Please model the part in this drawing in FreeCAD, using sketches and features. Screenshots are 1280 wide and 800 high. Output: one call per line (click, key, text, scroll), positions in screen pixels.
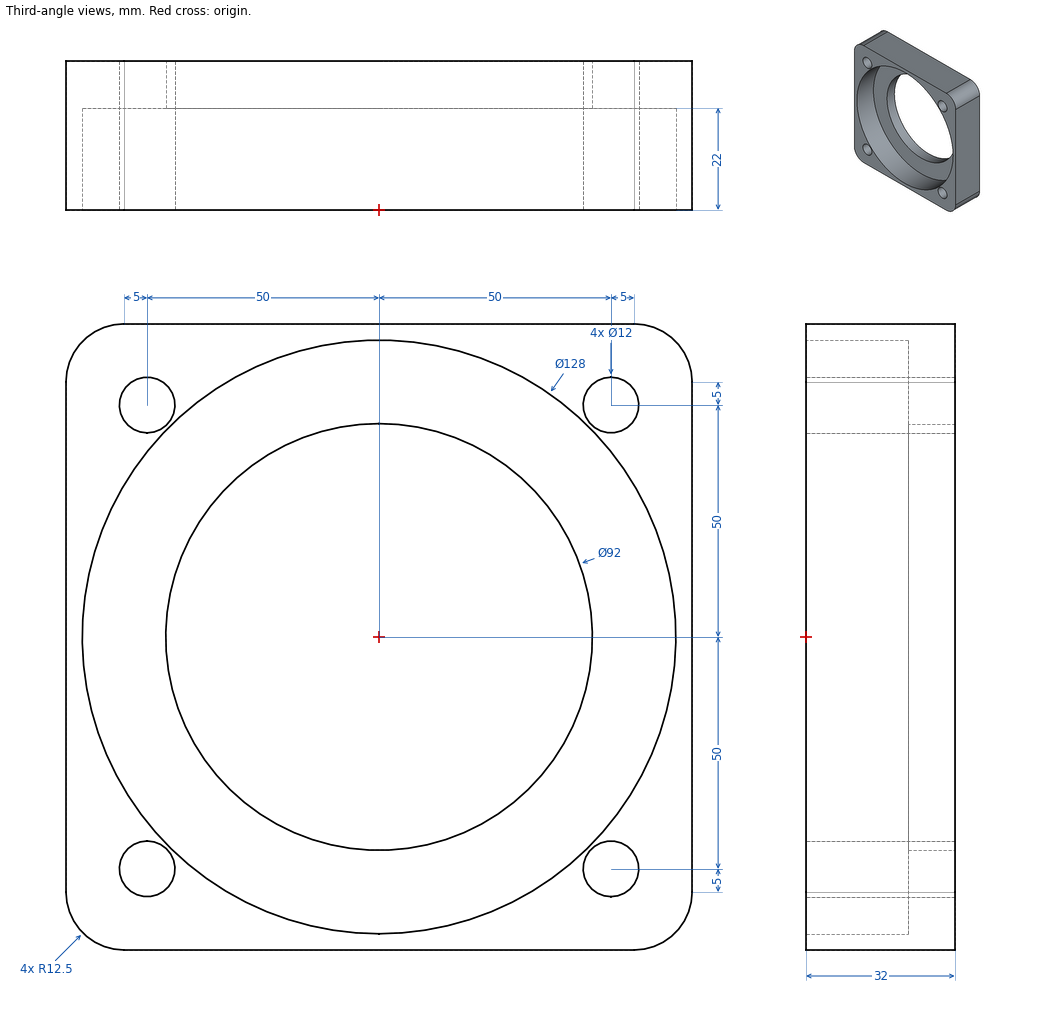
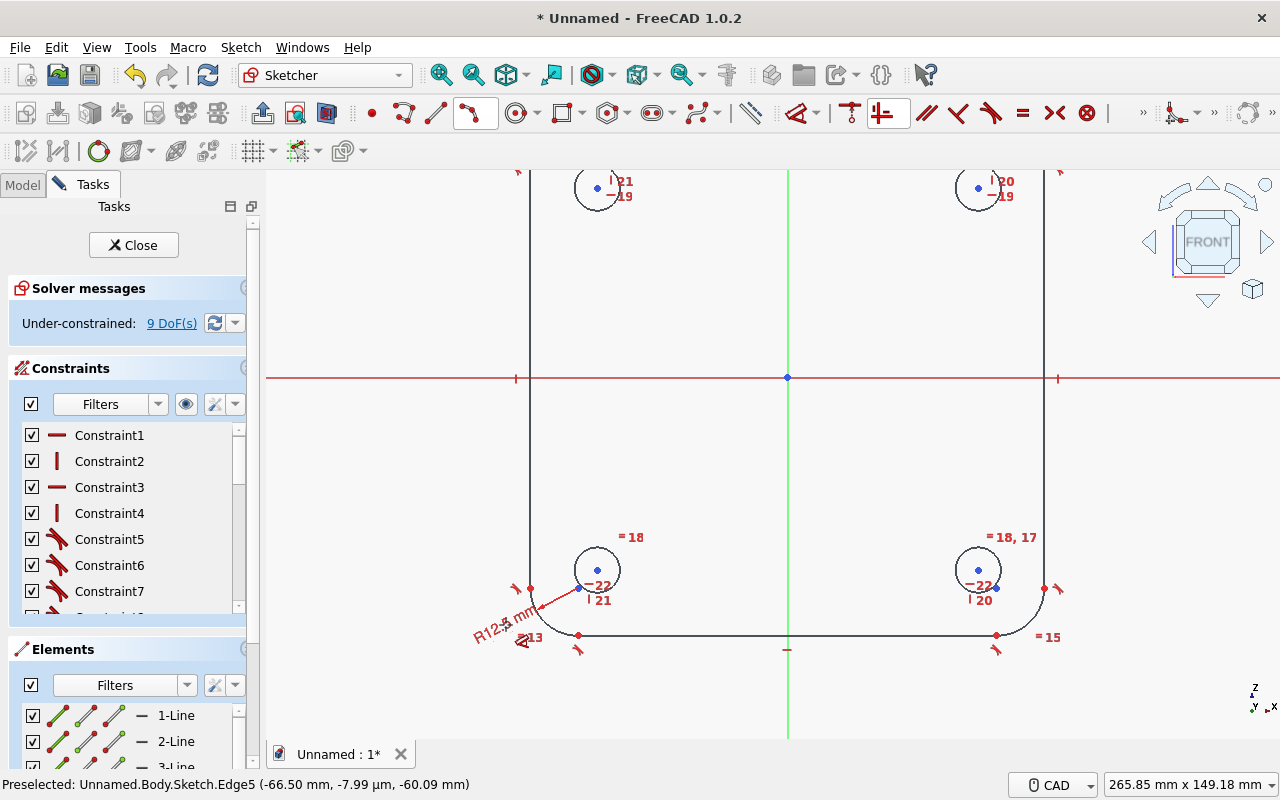
click(962, 204)
click(939, 226)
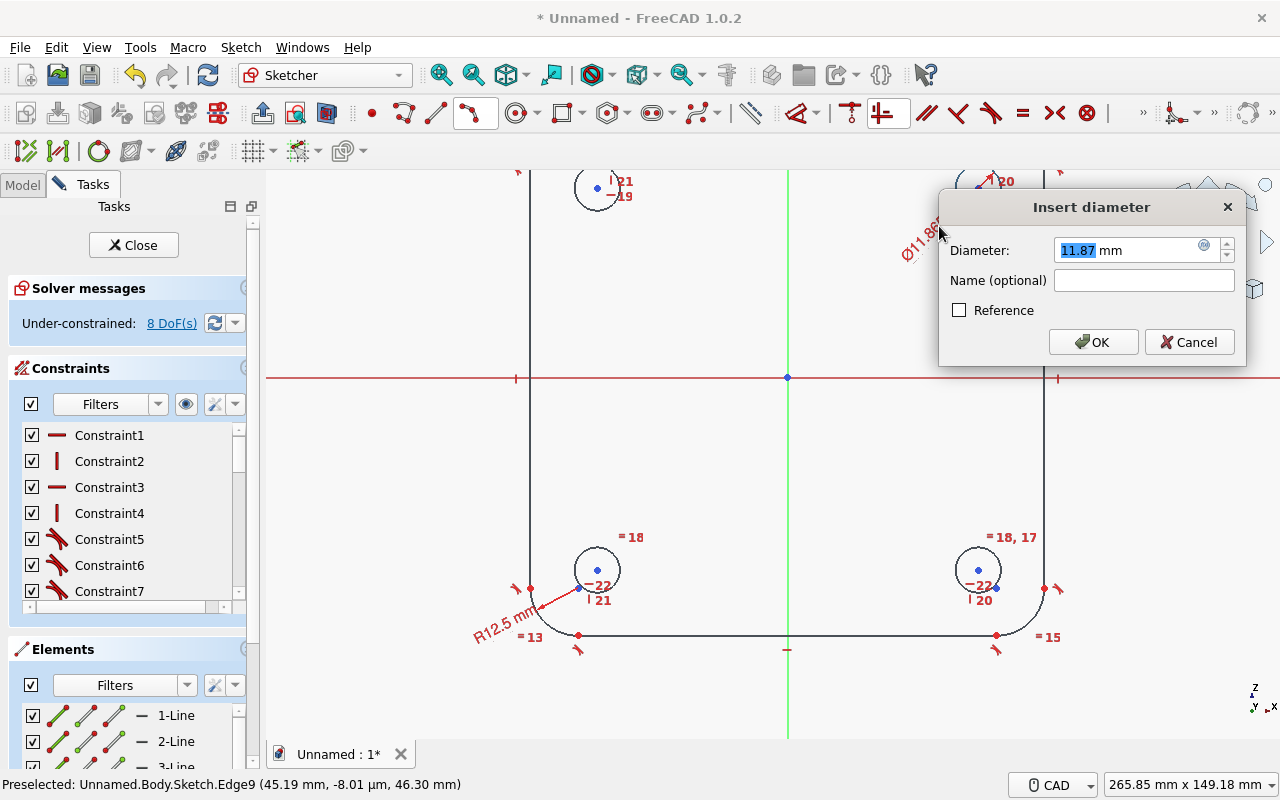
text(12)
key(Return)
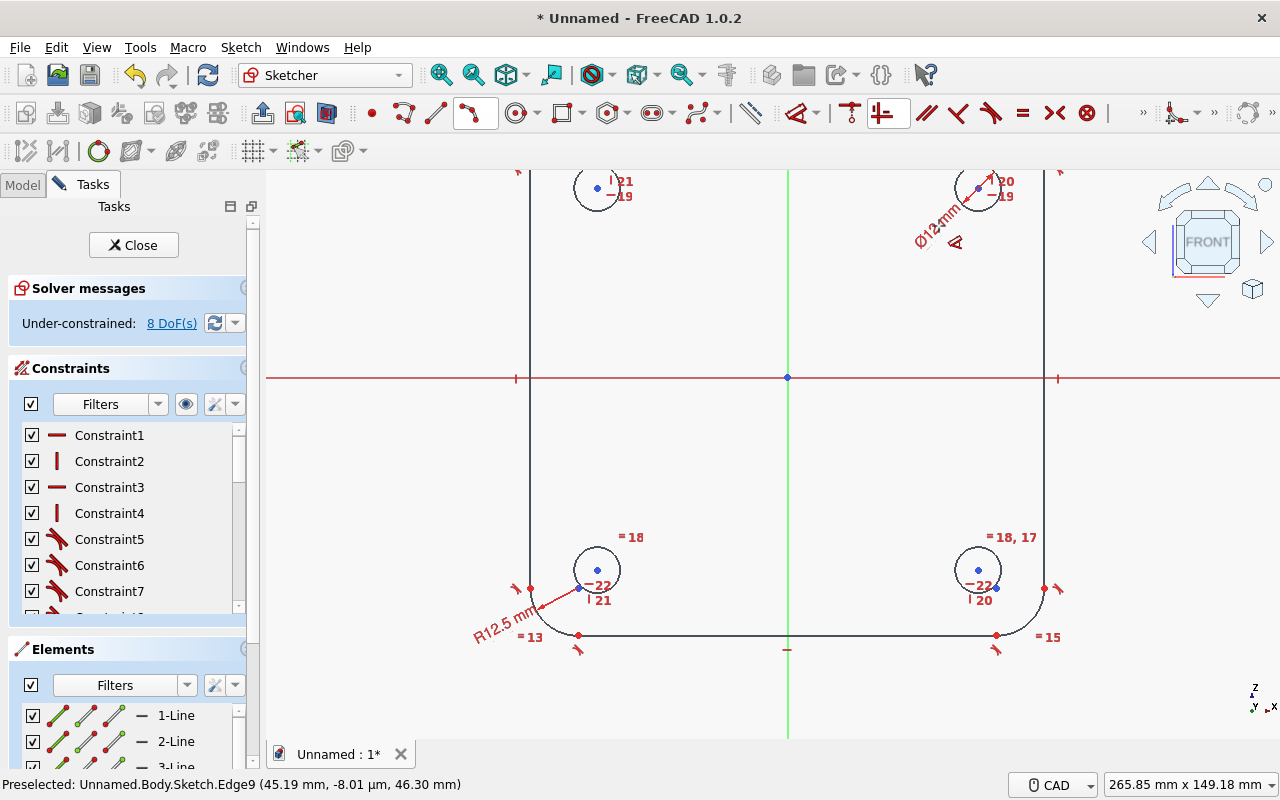
scroll(536, 610, down, 2)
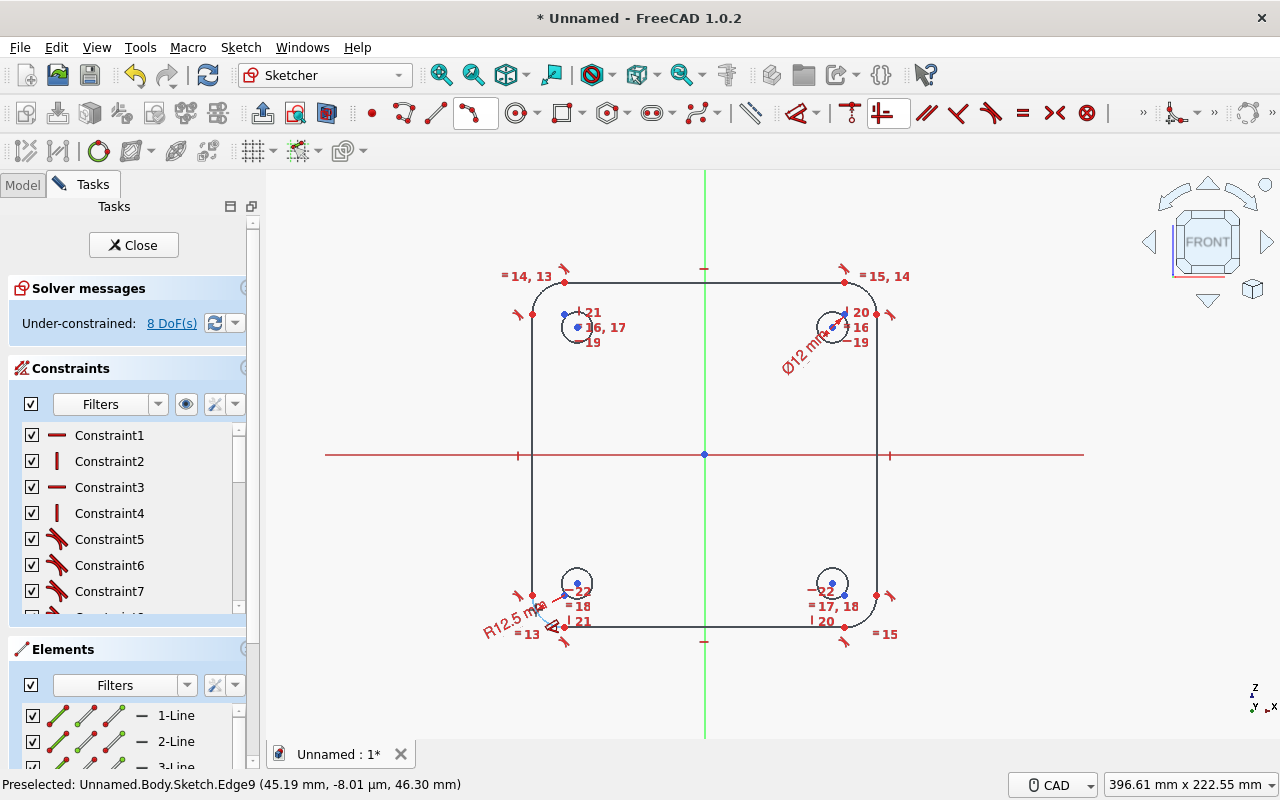
click(833, 327)
click(769, 489)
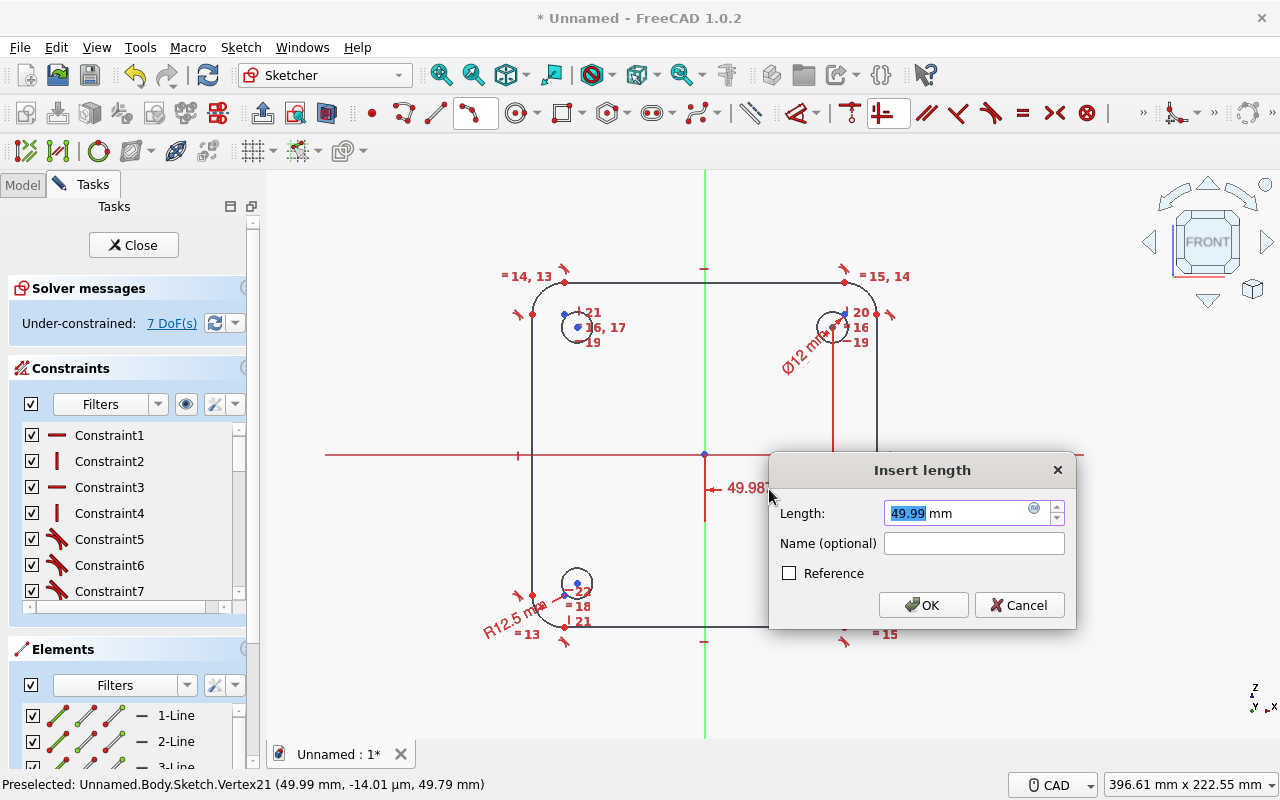
text(50)
key(Return)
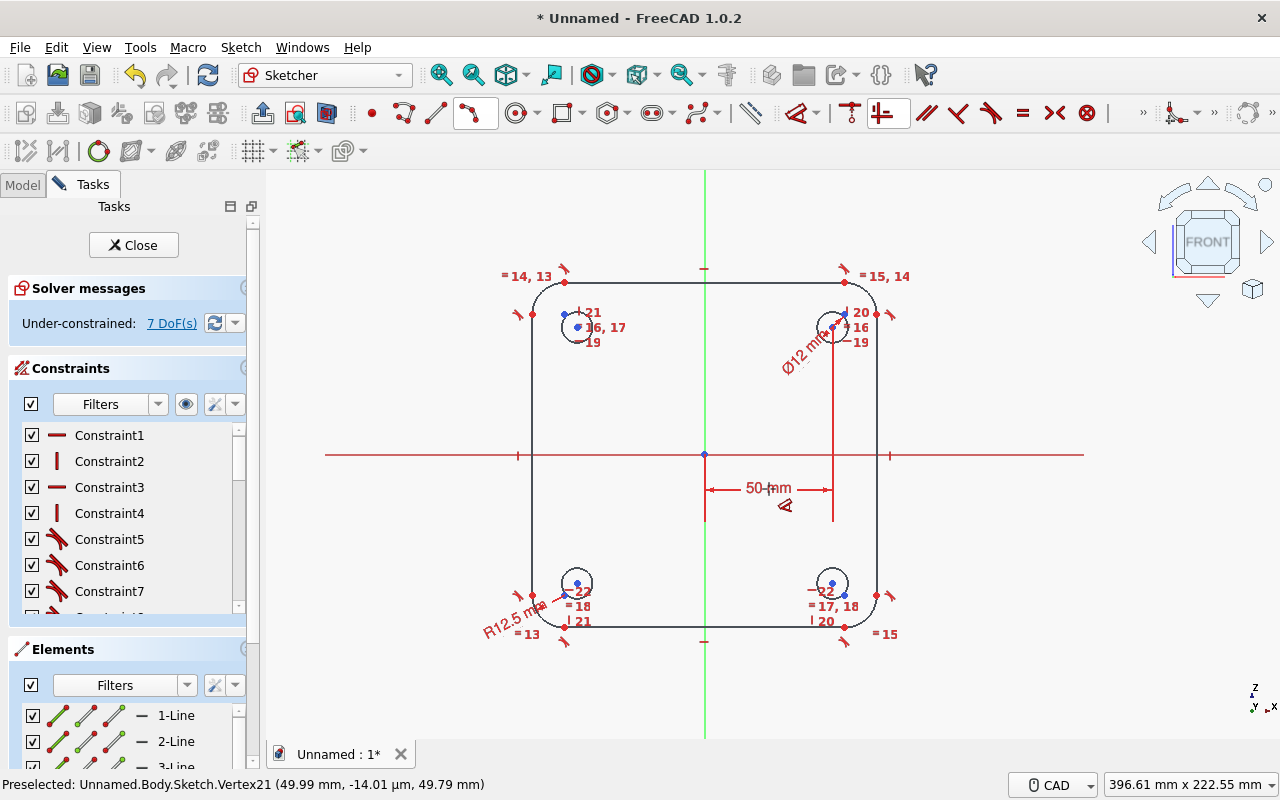
click(833, 327)
click(671, 391)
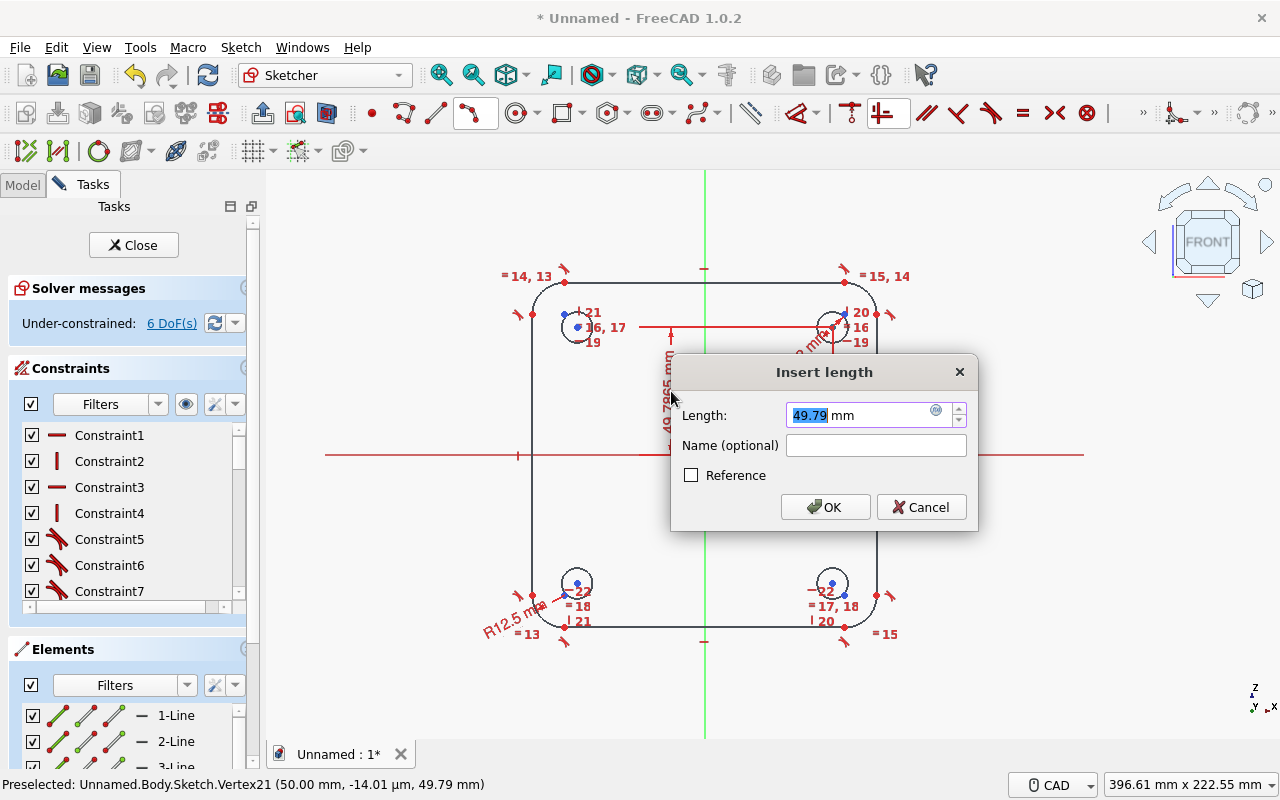
text(50)
key(Return)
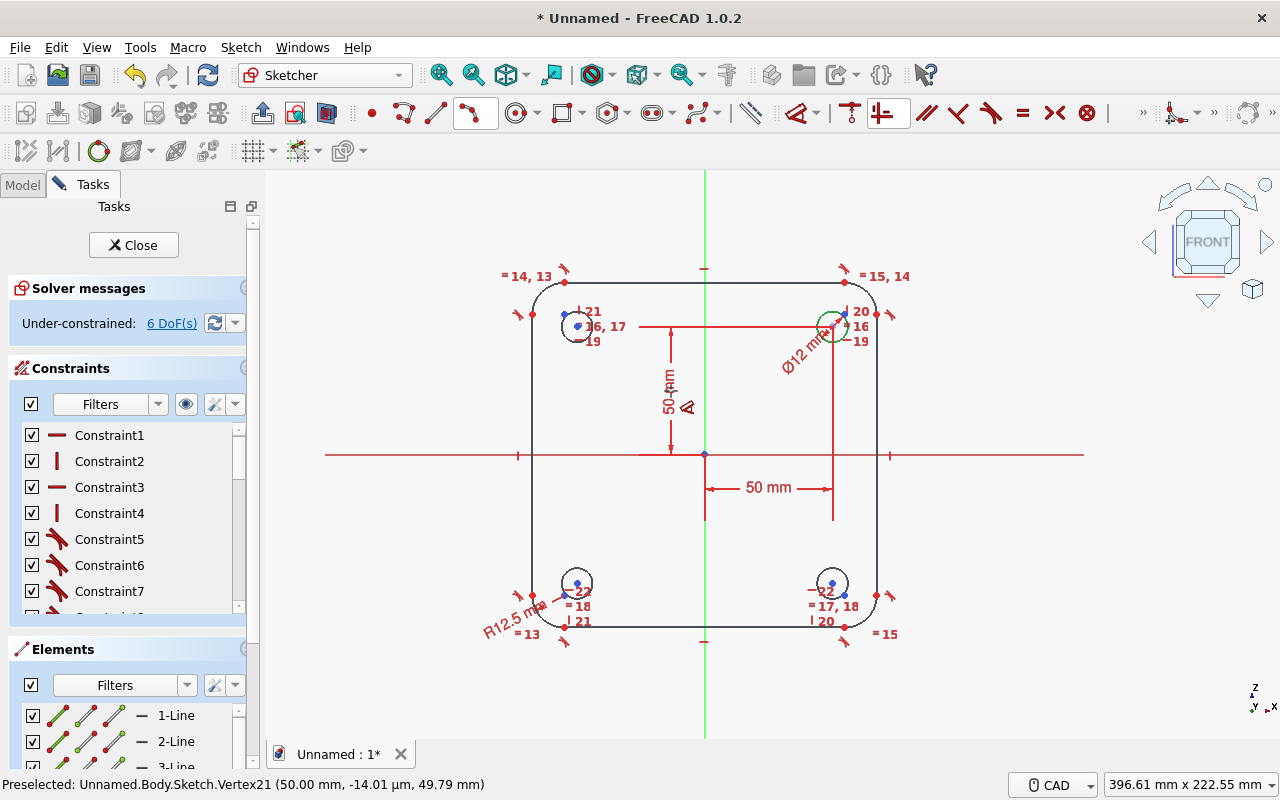
click(577, 327)
click(641, 489)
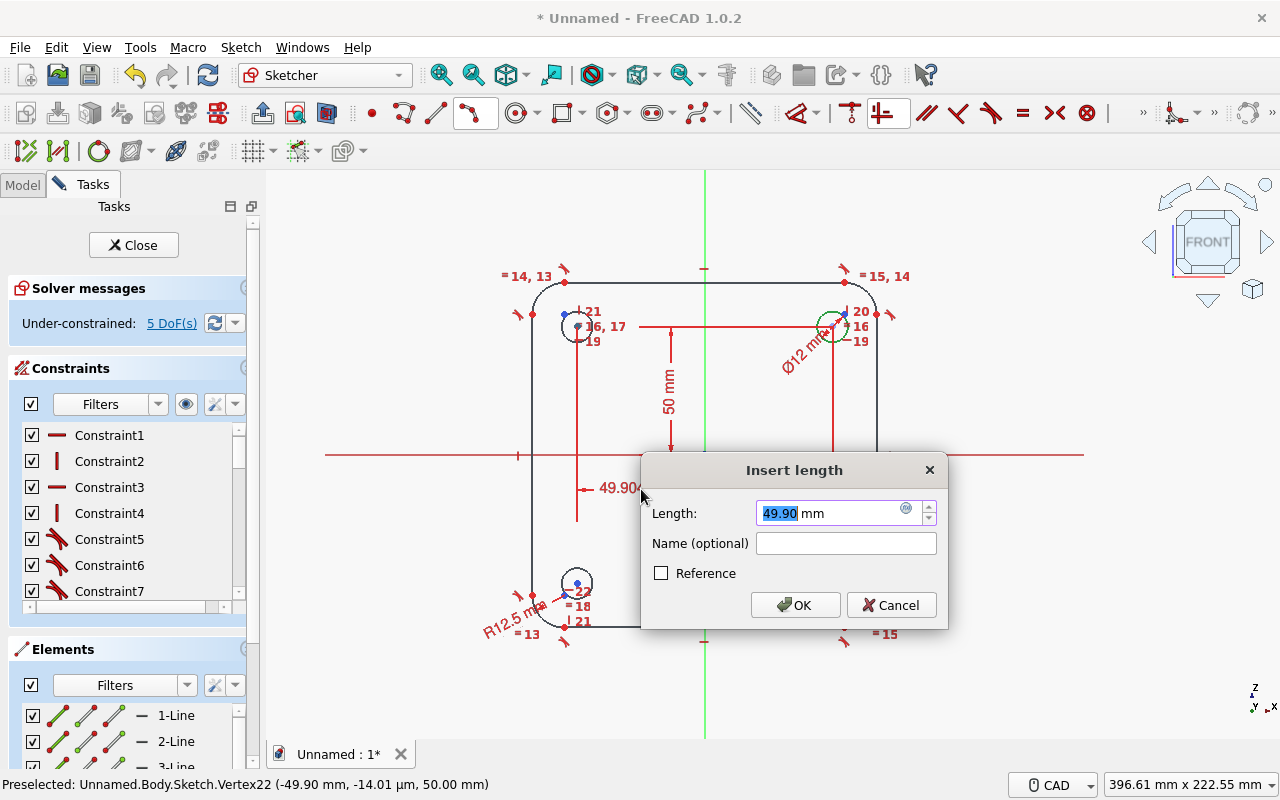
text(50)
key(Return)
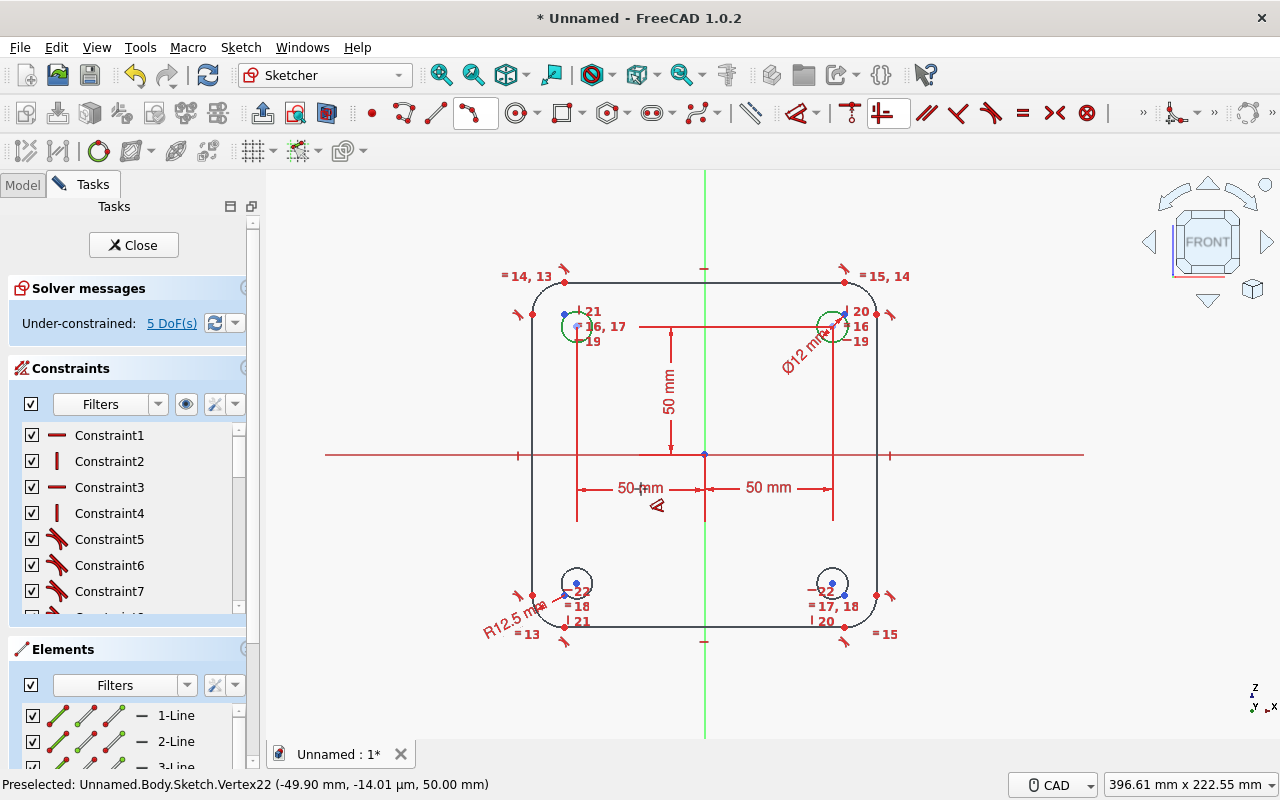
click(833, 583)
click(671, 519)